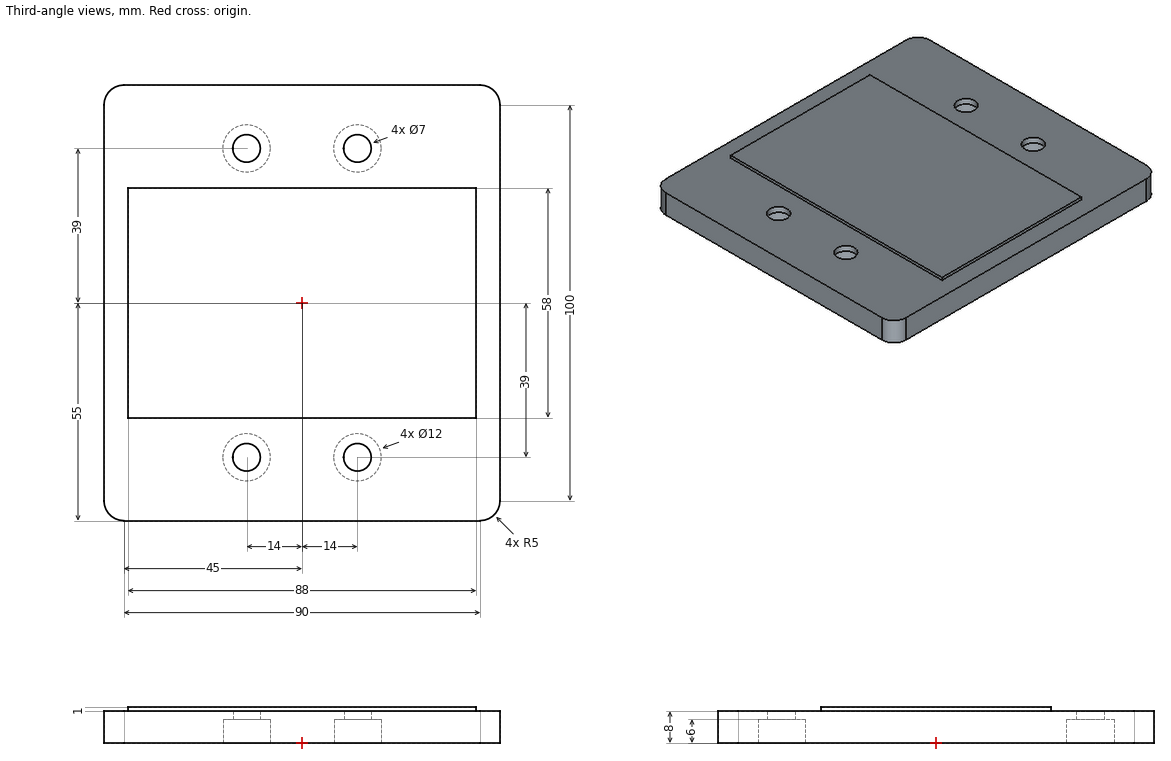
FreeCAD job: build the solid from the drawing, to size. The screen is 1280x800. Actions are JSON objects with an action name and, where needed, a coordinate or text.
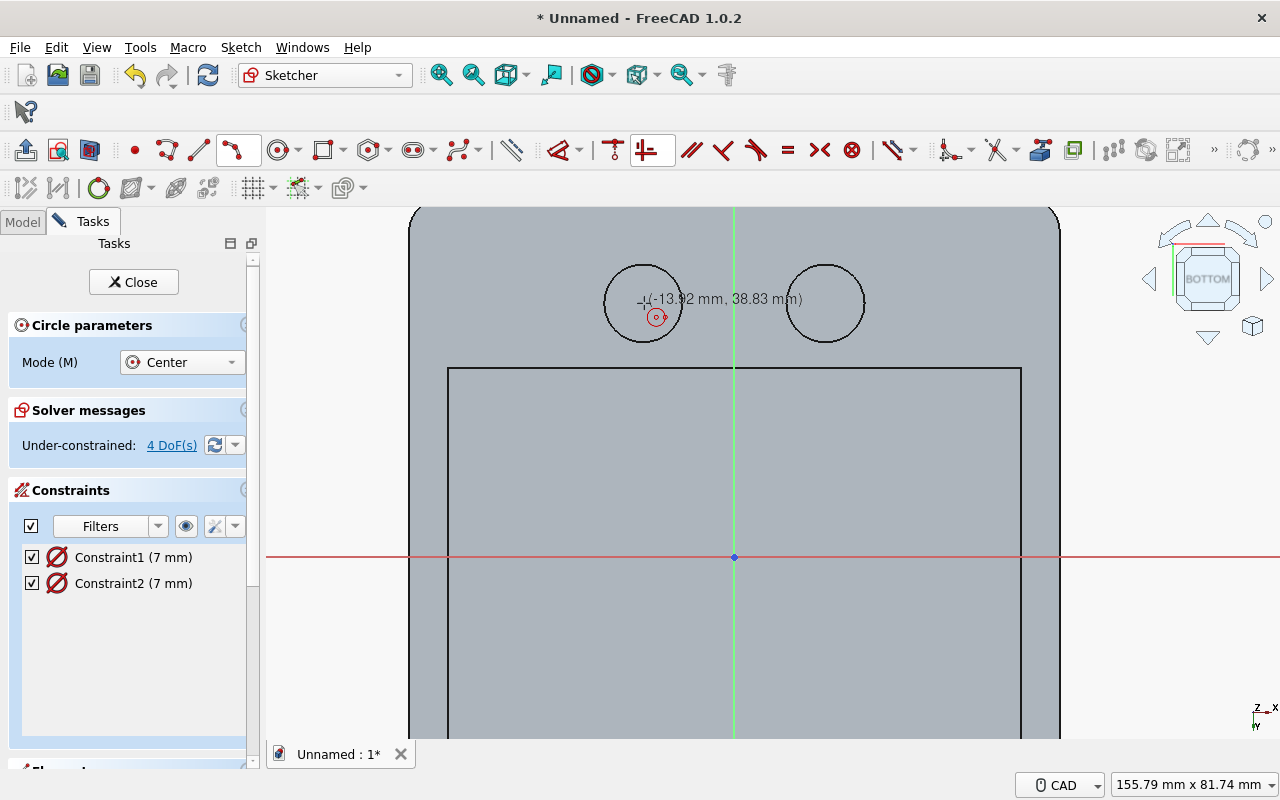
{"action": "left_click", "coordinate": [643, 303]}
{"action": "mouse_move", "coordinate": [659, 287]}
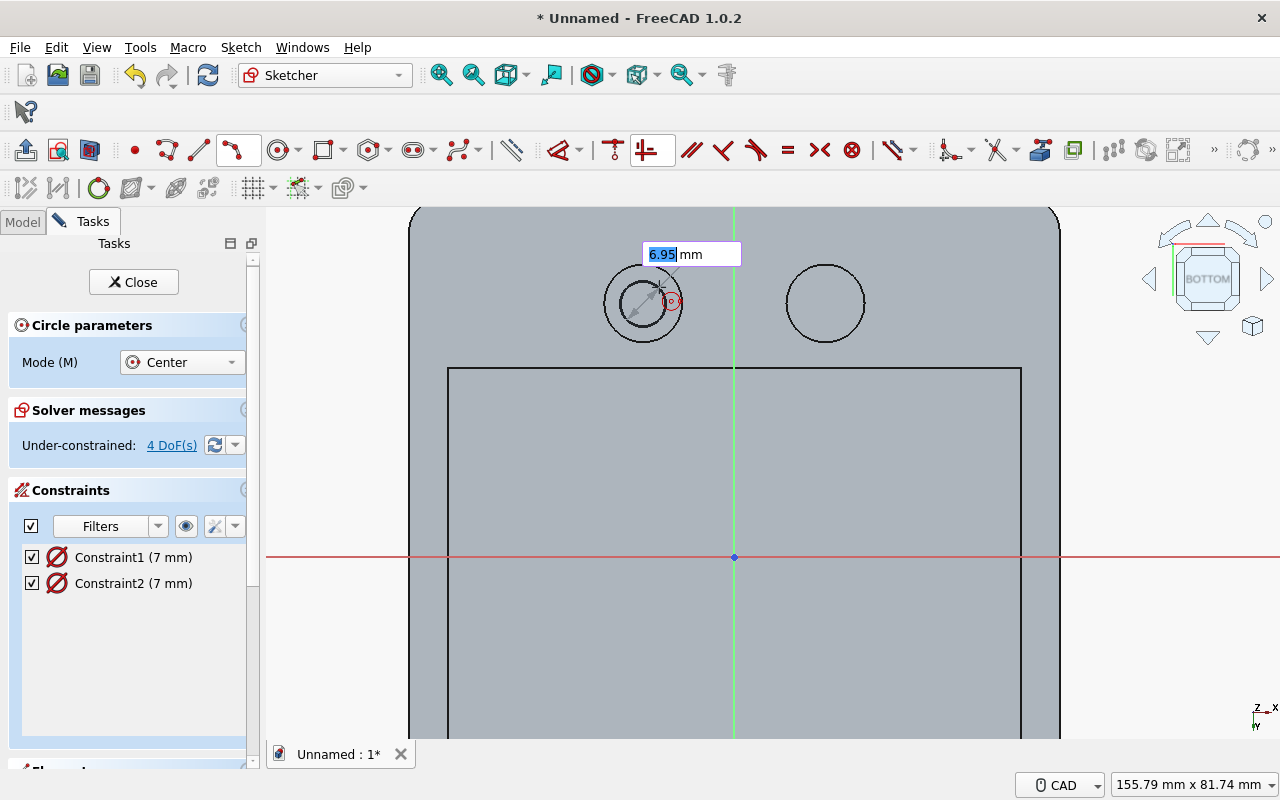
{"action": "type", "text": "7"}
{"action": "key", "text": "Return"}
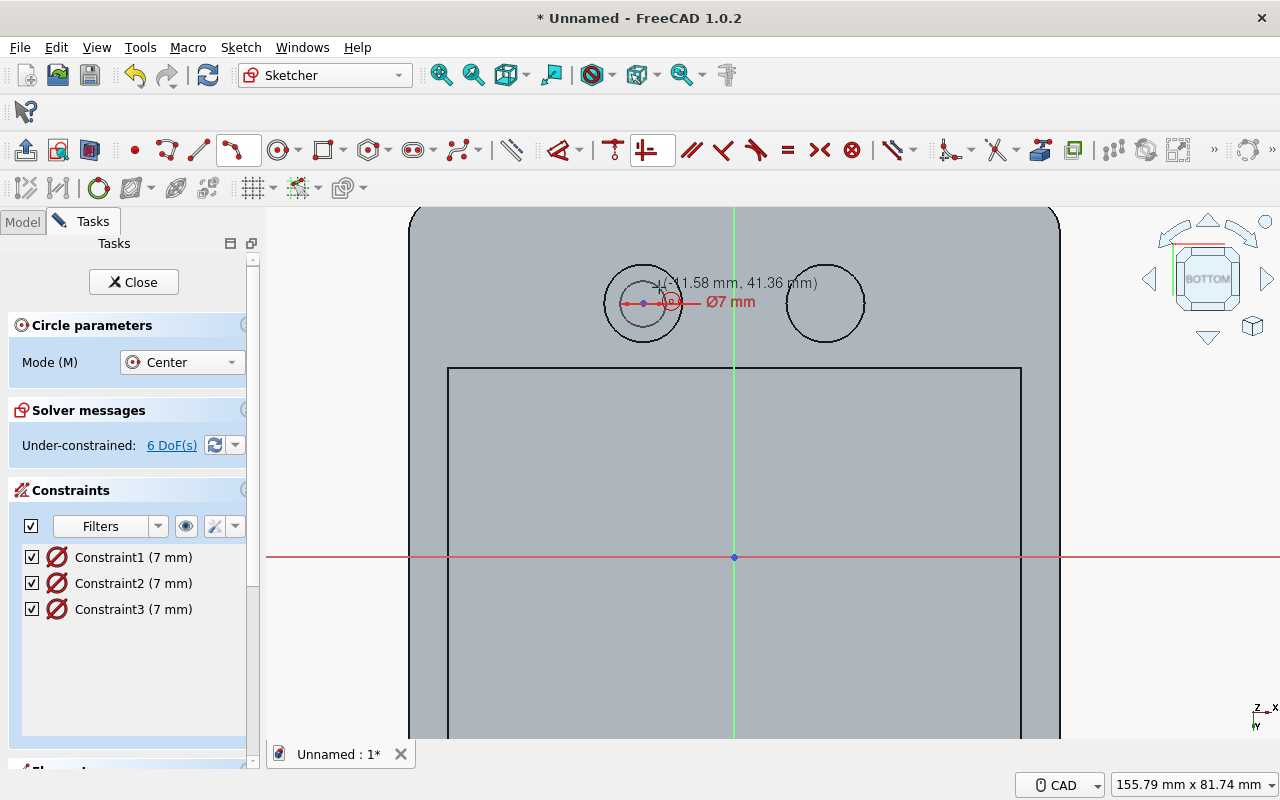
{"action": "left_click", "coordinate": [826, 303]}
{"action": "mouse_move", "coordinate": [842, 287]}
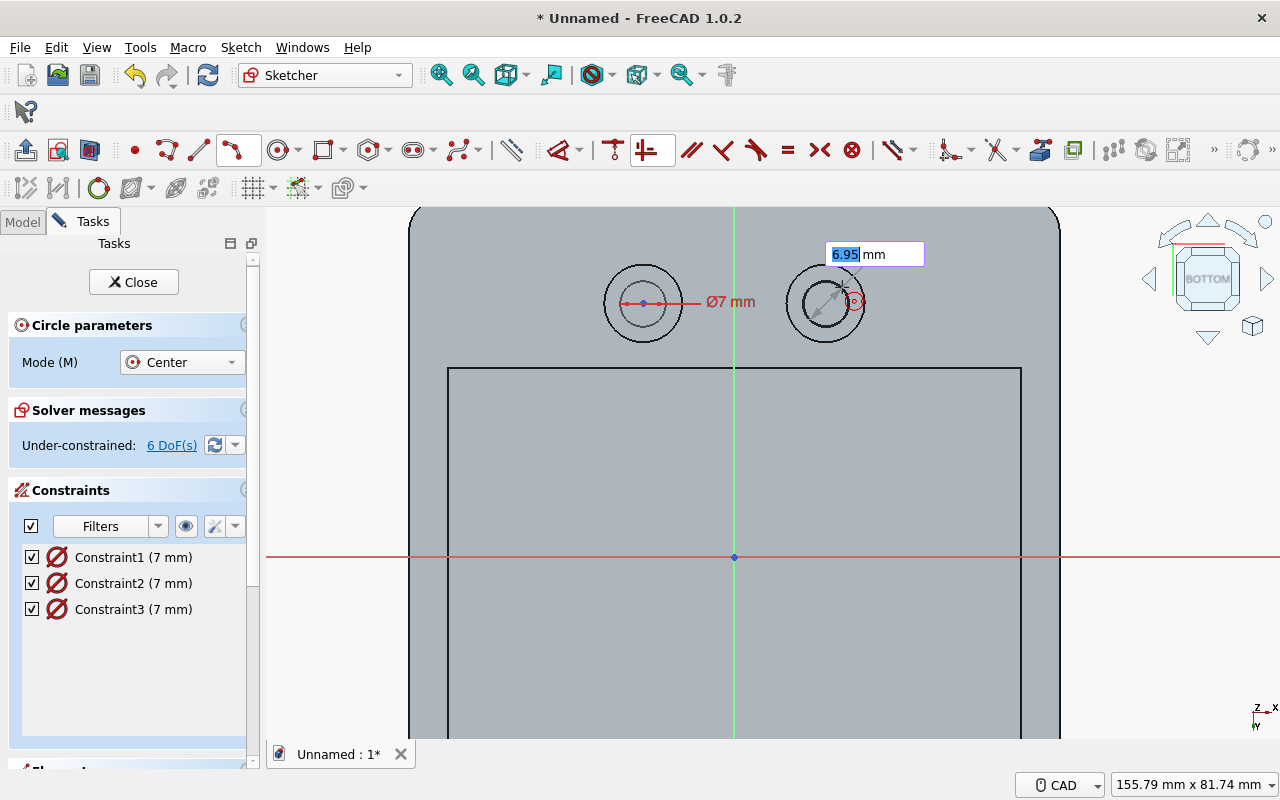
{"action": "type", "text": "7"}
{"action": "key", "text": "Return"}
{"action": "key", "text": "Escape"}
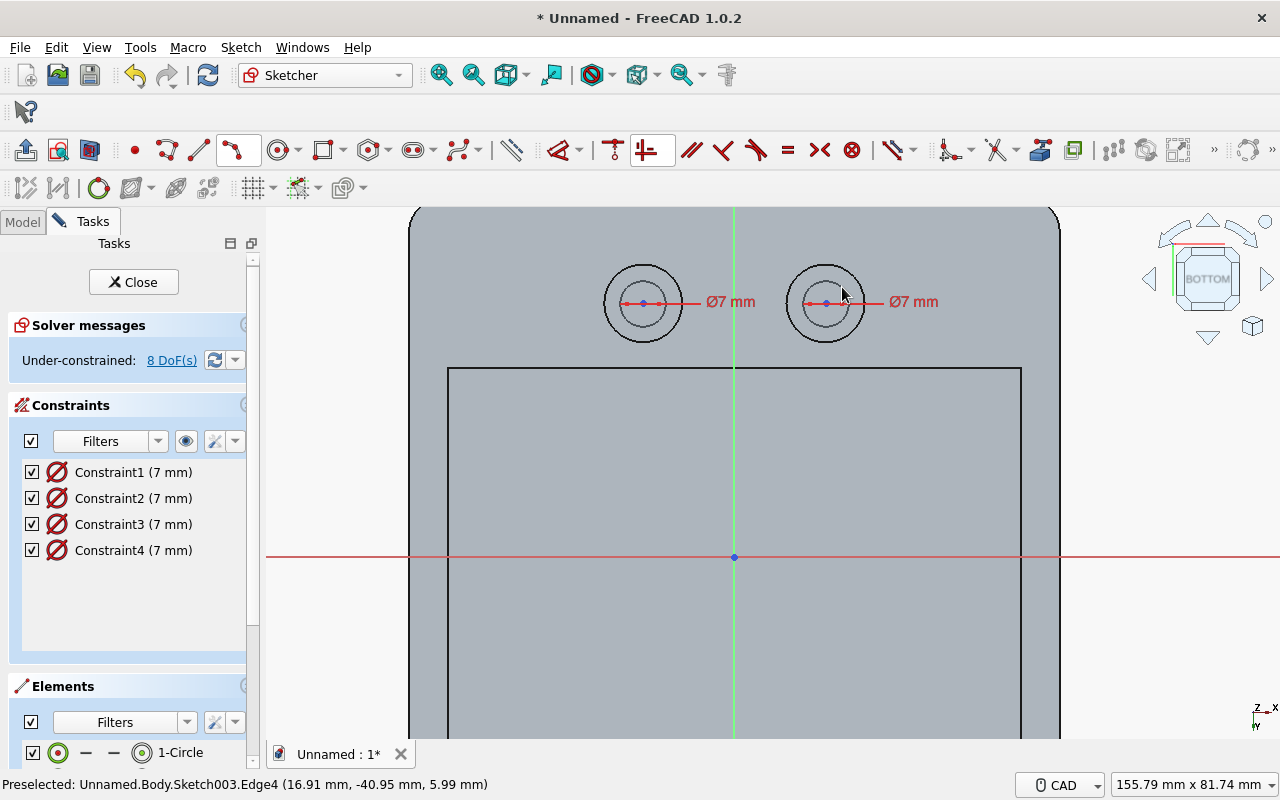
{"action": "scroll", "coordinate": [644, 302], "scroll_direction": "down", "scroll_amount": 2}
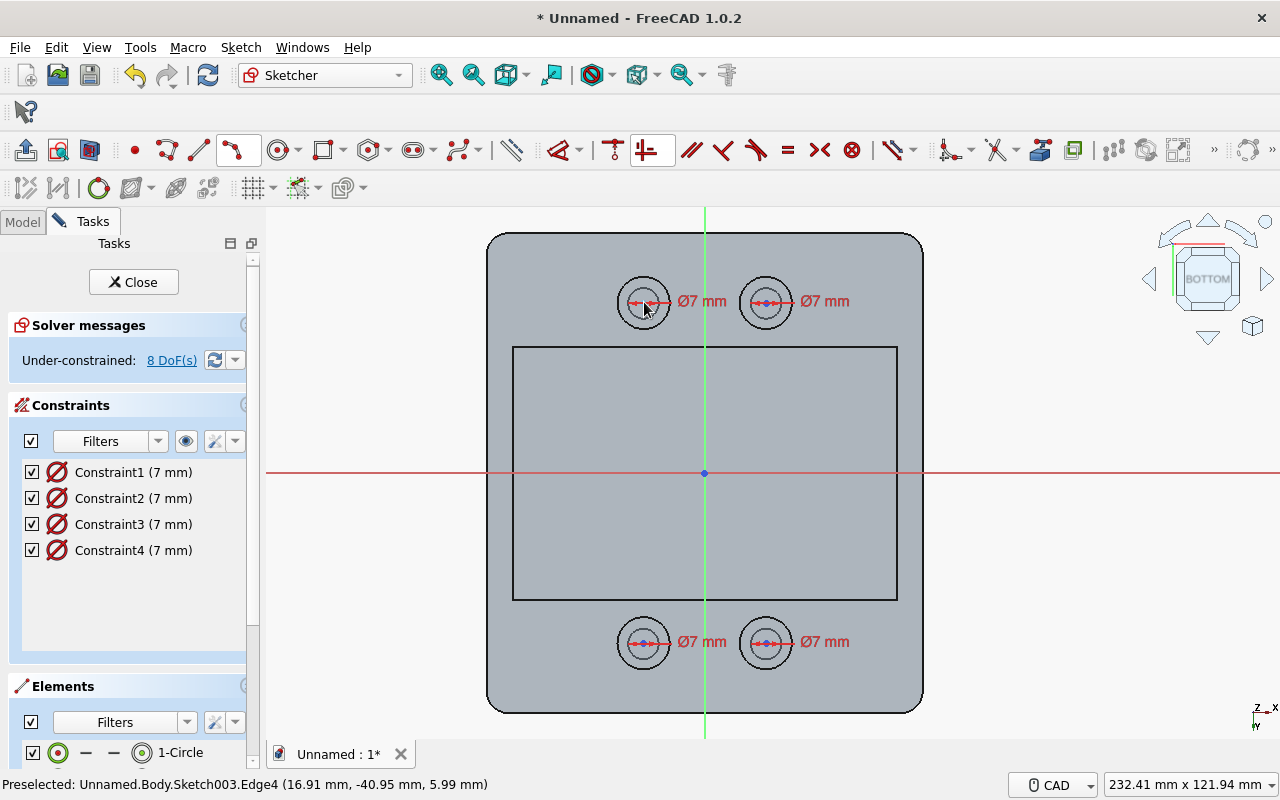
{"action": "left_click", "coordinate": [766, 644]}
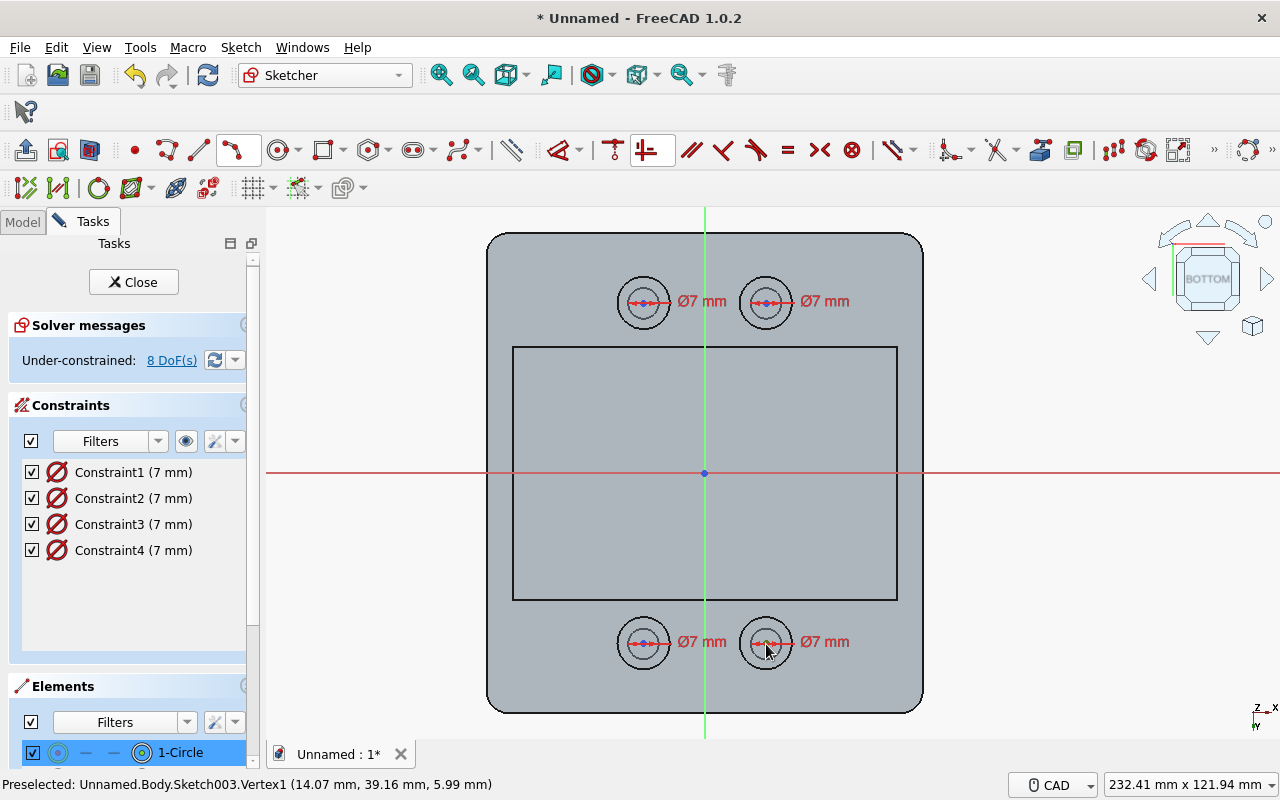
{"action": "left_click", "coordinate": [643, 644]}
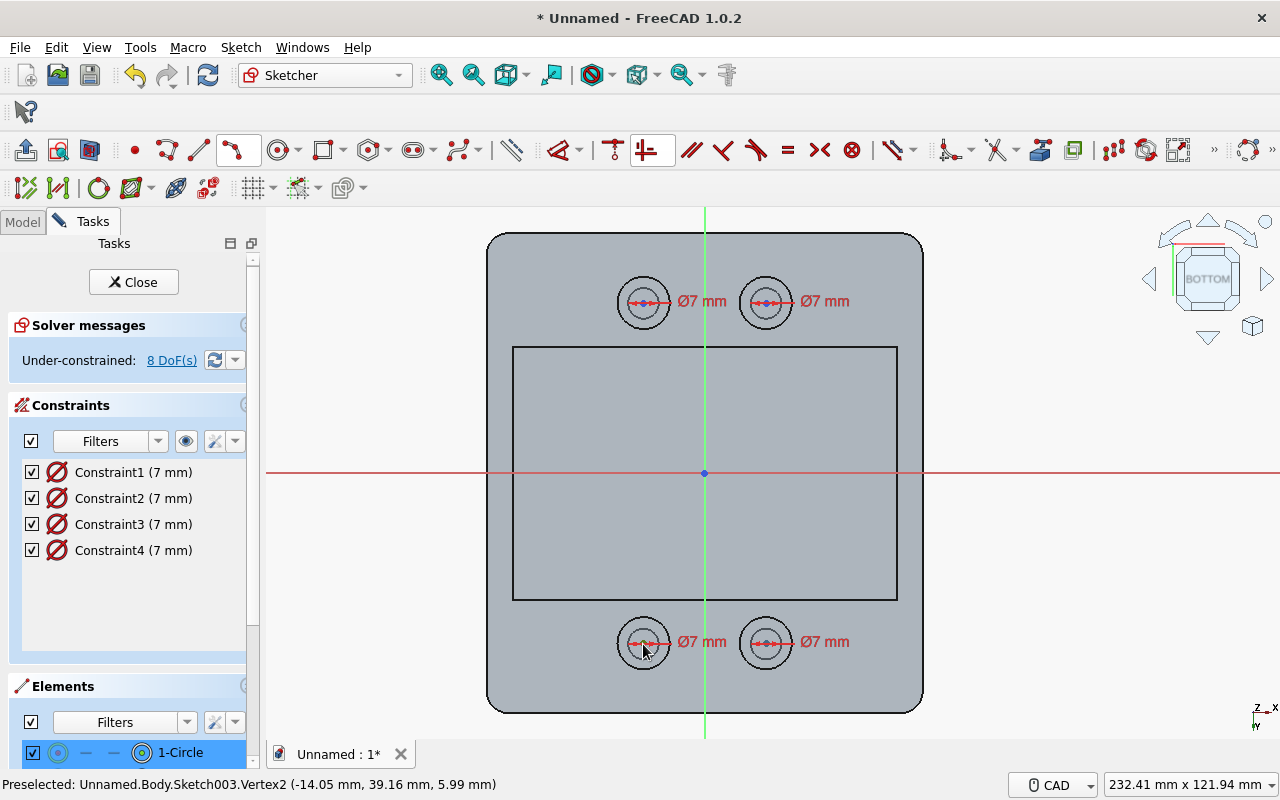
{"action": "key", "text": "h"}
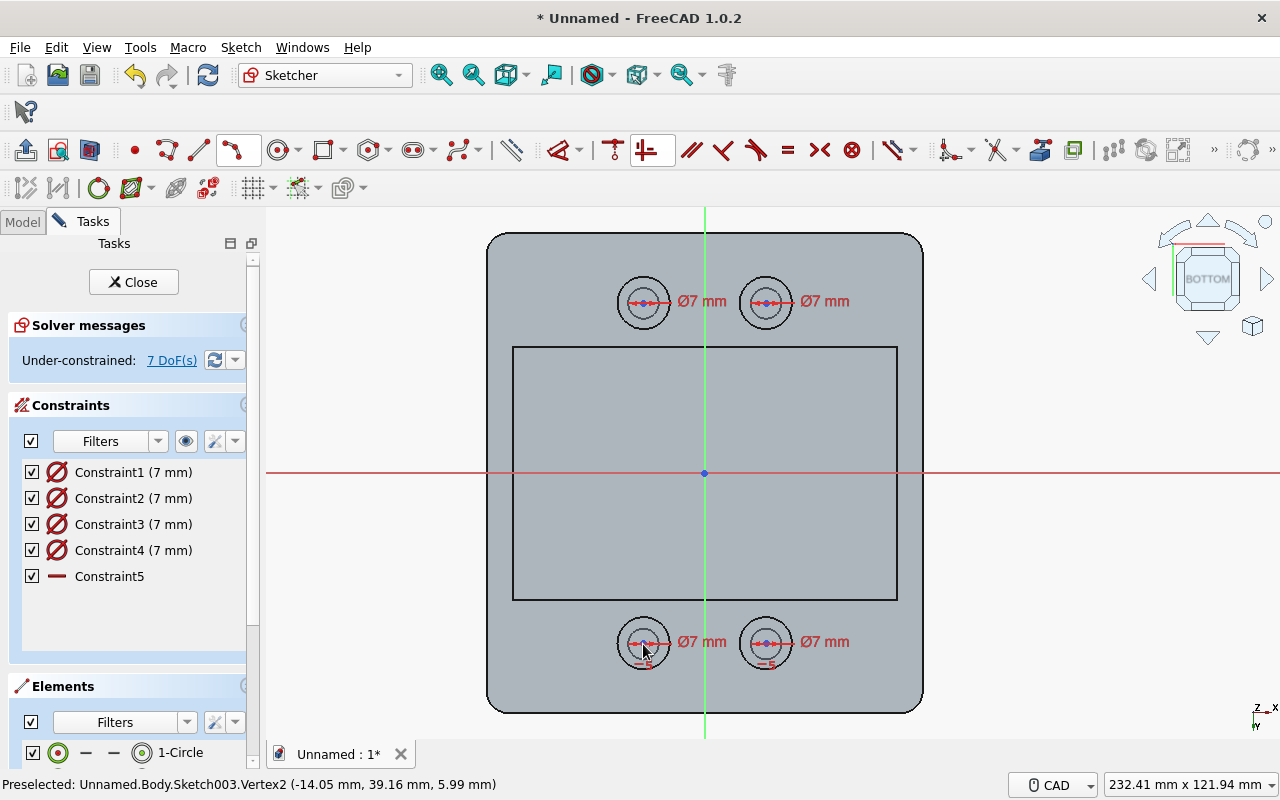
{"action": "left_click", "coordinate": [643, 644]}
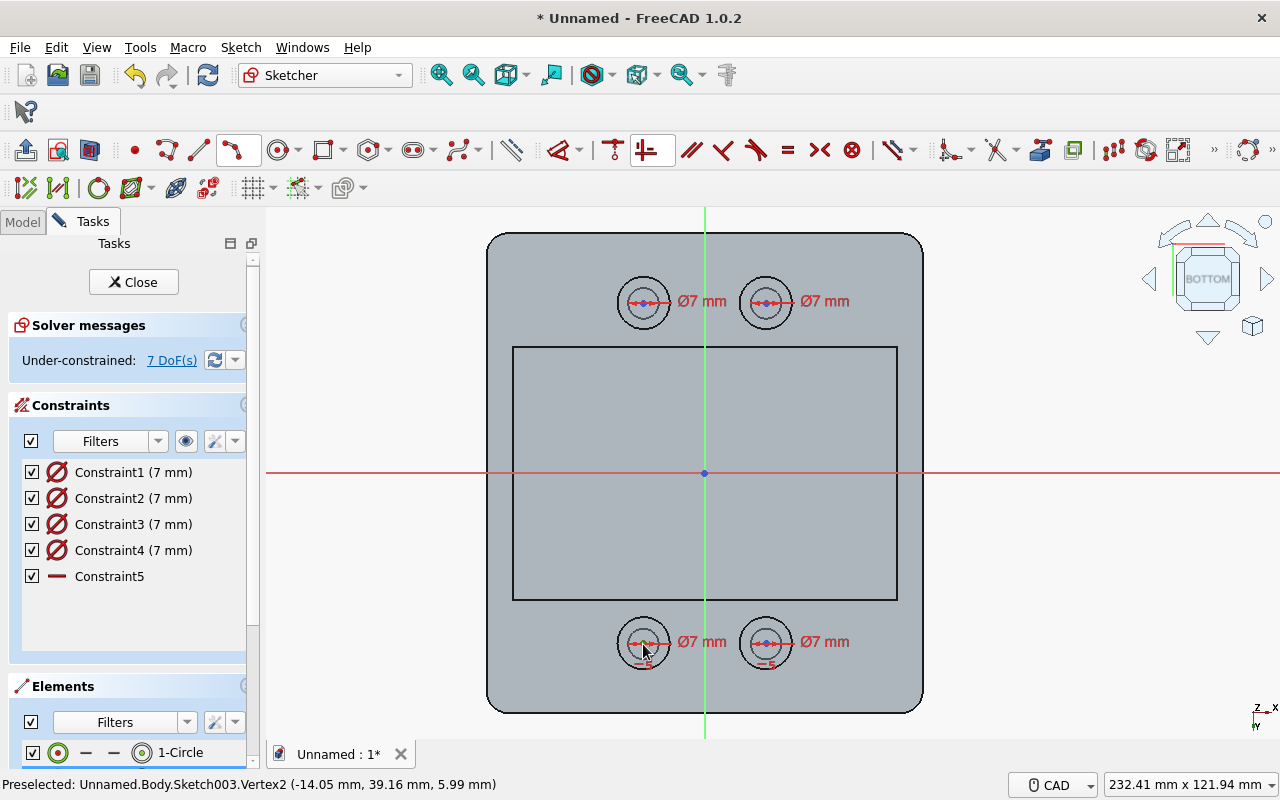
{"action": "left_click", "coordinate": [643, 303]}